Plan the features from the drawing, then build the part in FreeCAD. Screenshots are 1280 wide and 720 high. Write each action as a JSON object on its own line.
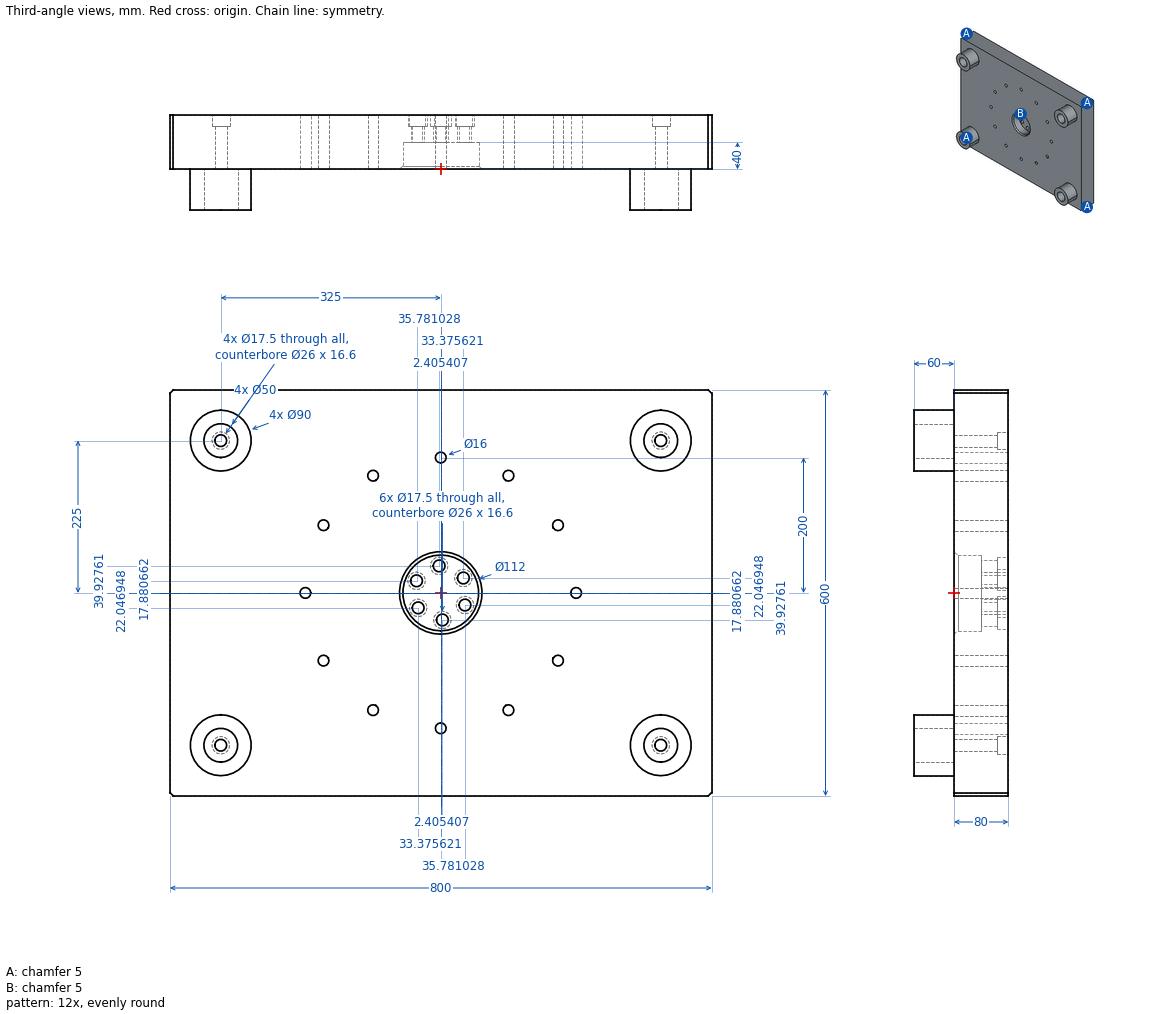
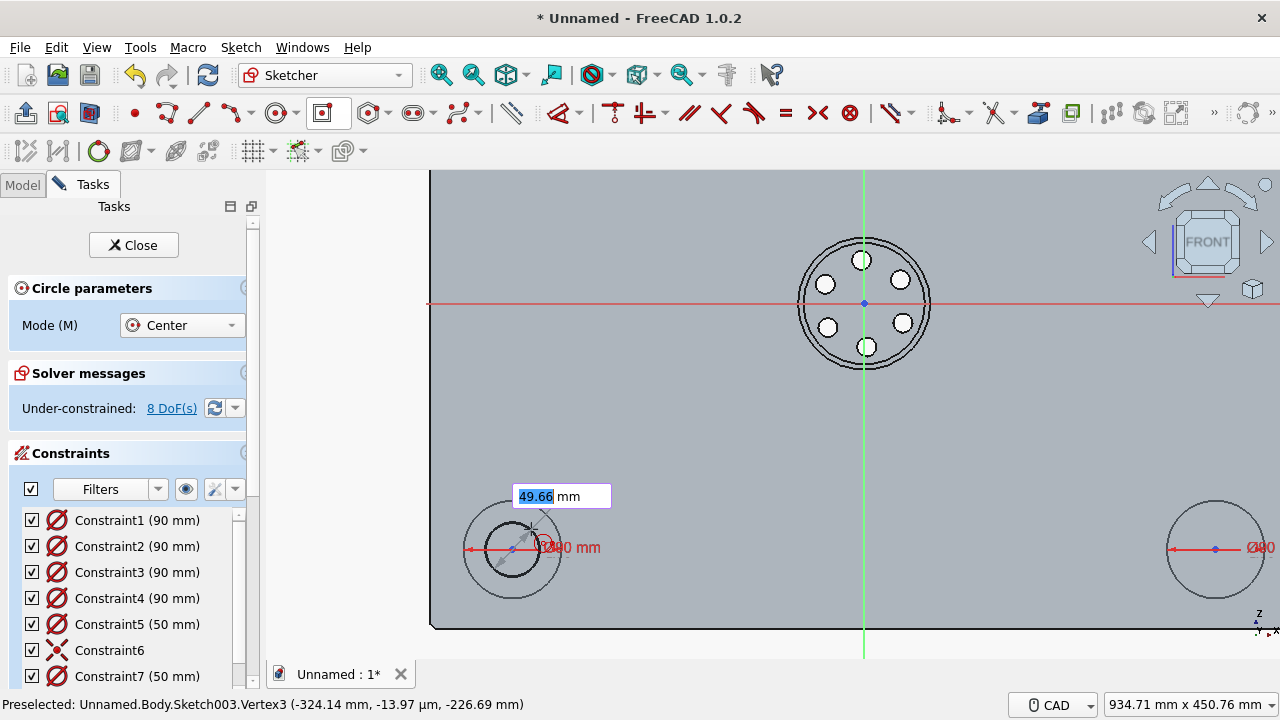
{"action": "type", "text": "50"}
{"action": "key", "text": "Return"}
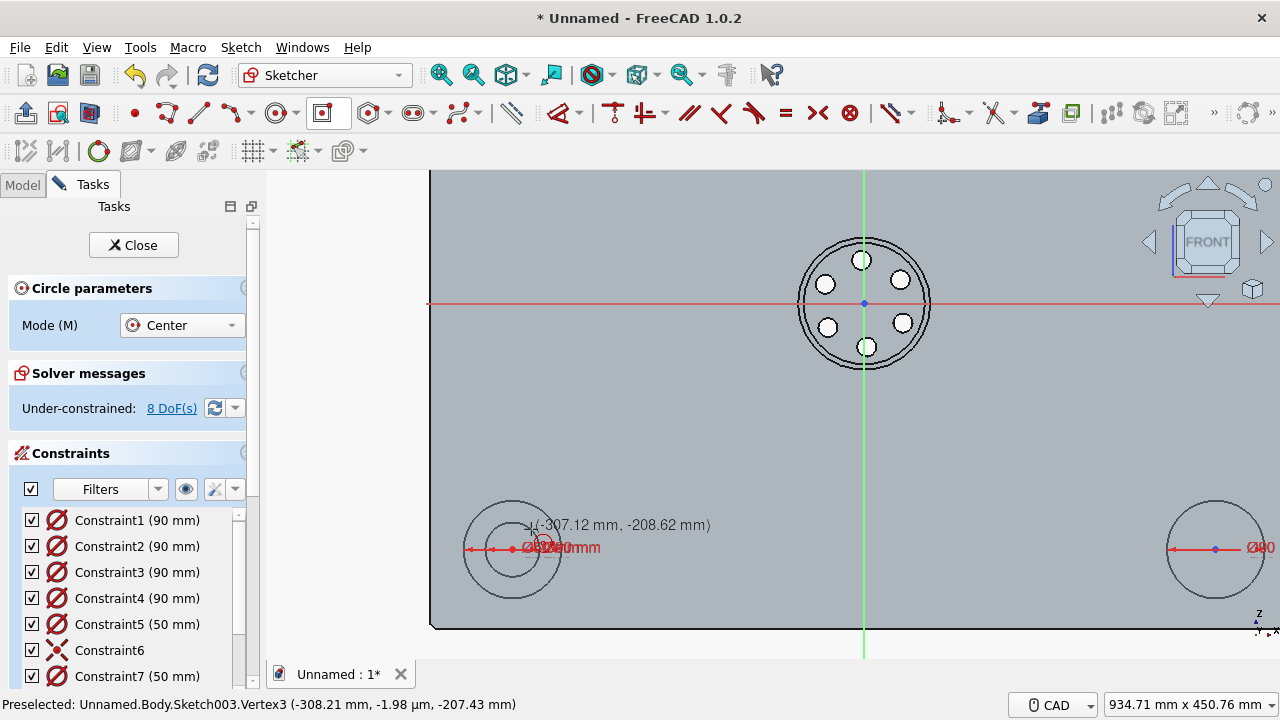
{"action": "scroll", "coordinate": [510, 549], "scroll_direction": "down", "scroll_amount": 3}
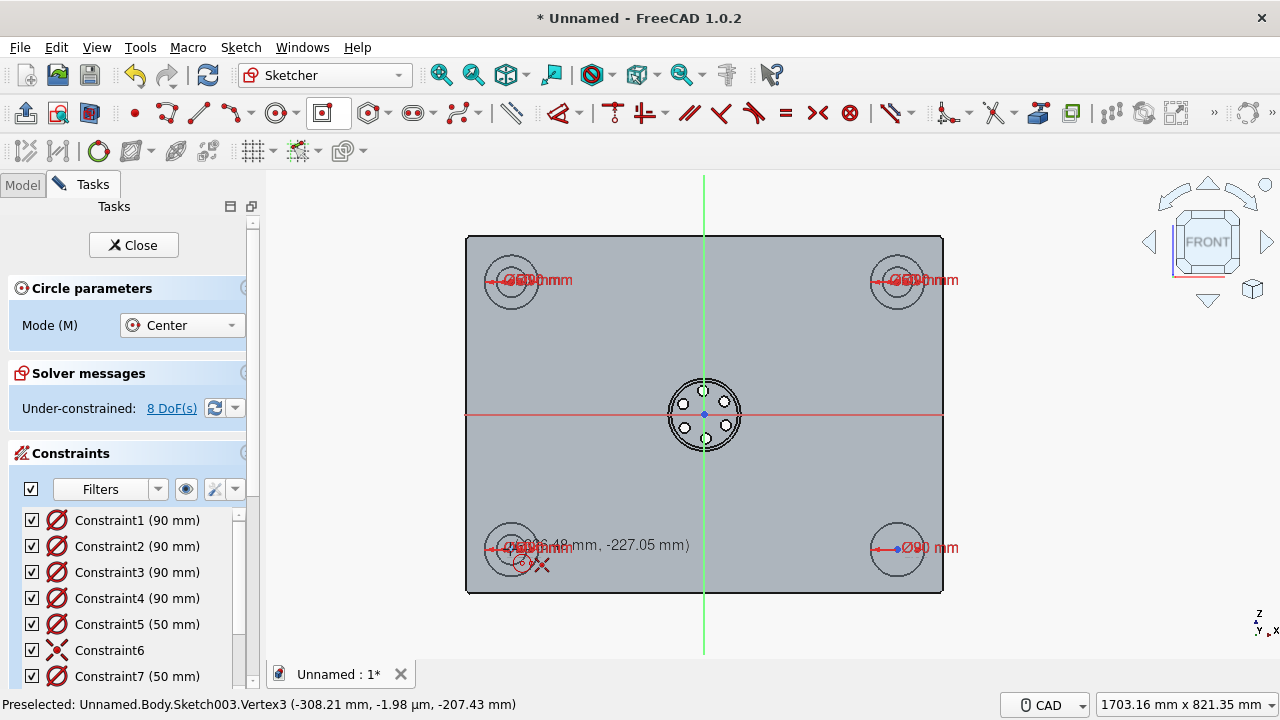
{"action": "scroll", "coordinate": [898, 549], "scroll_direction": "up", "scroll_amount": 3}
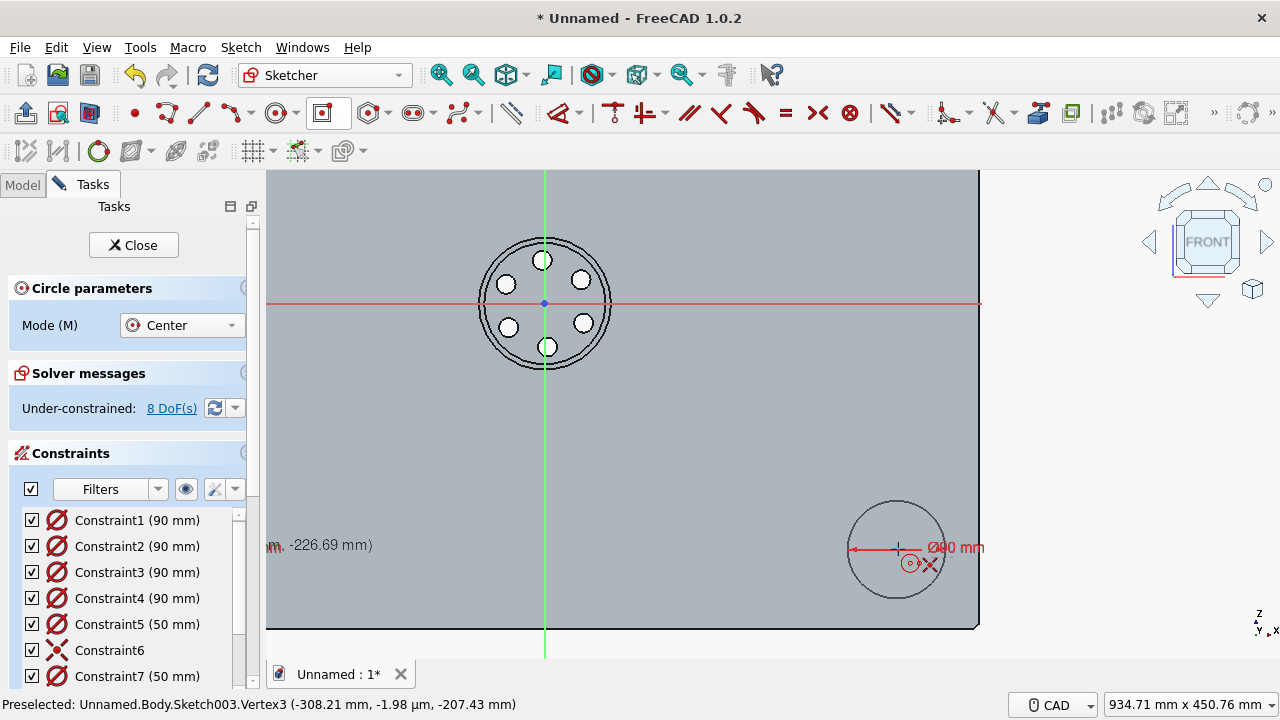
{"action": "left_click", "coordinate": [897, 550]}
{"action": "mouse_move", "coordinate": [917, 529]}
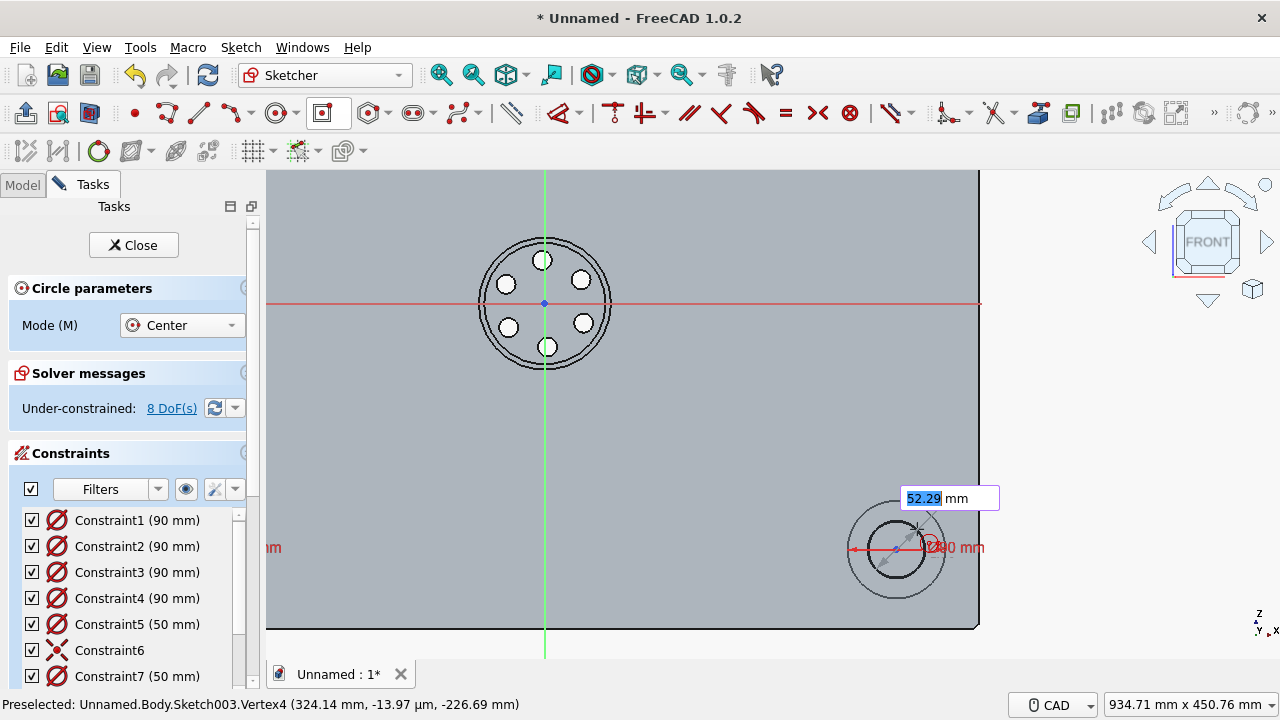
{"action": "type", "text": "50"}
{"action": "key", "text": "Return"}
{"action": "key", "text": "Escape"}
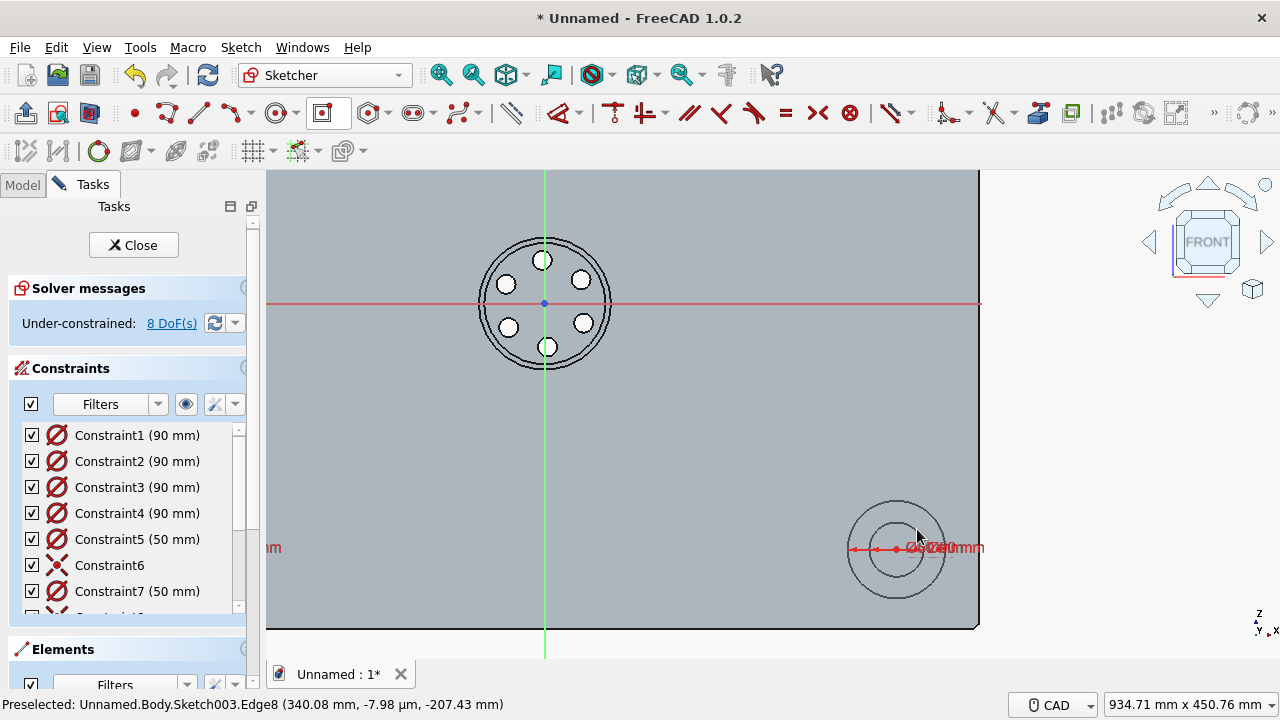
{"action": "scroll", "coordinate": [899, 549], "scroll_direction": "down", "scroll_amount": 3}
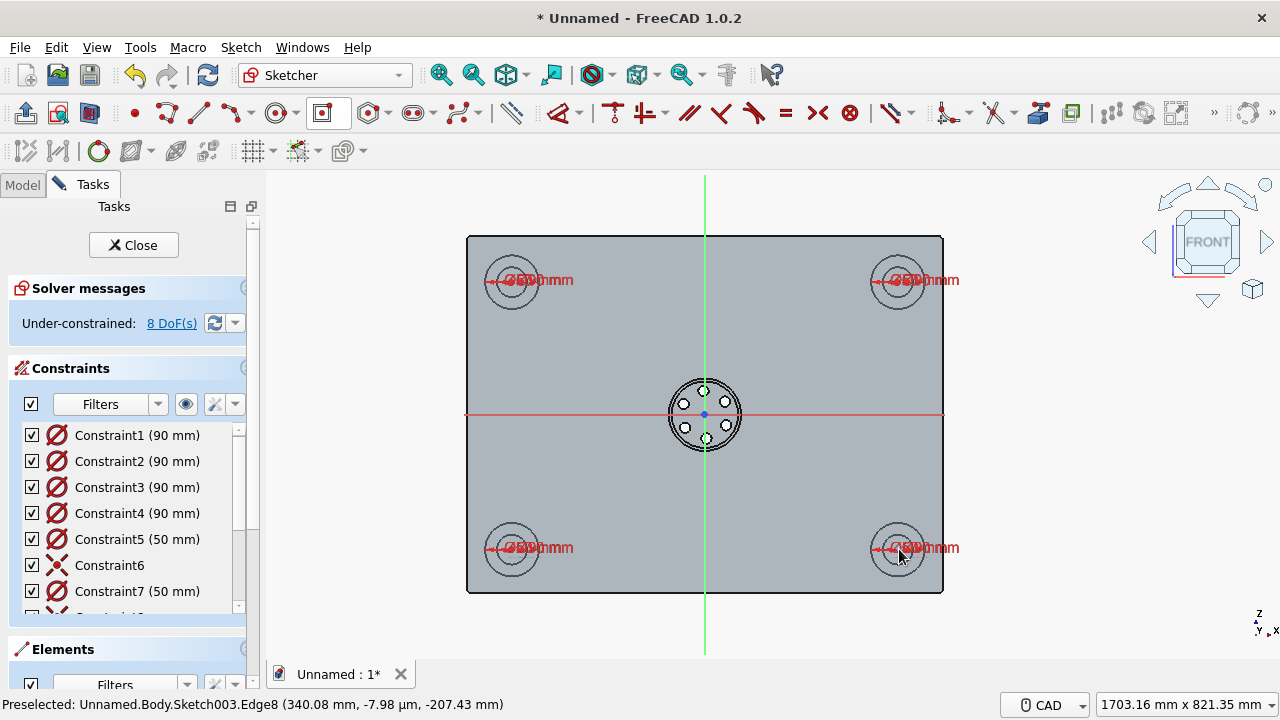
{"action": "left_click", "coordinate": [512, 282]}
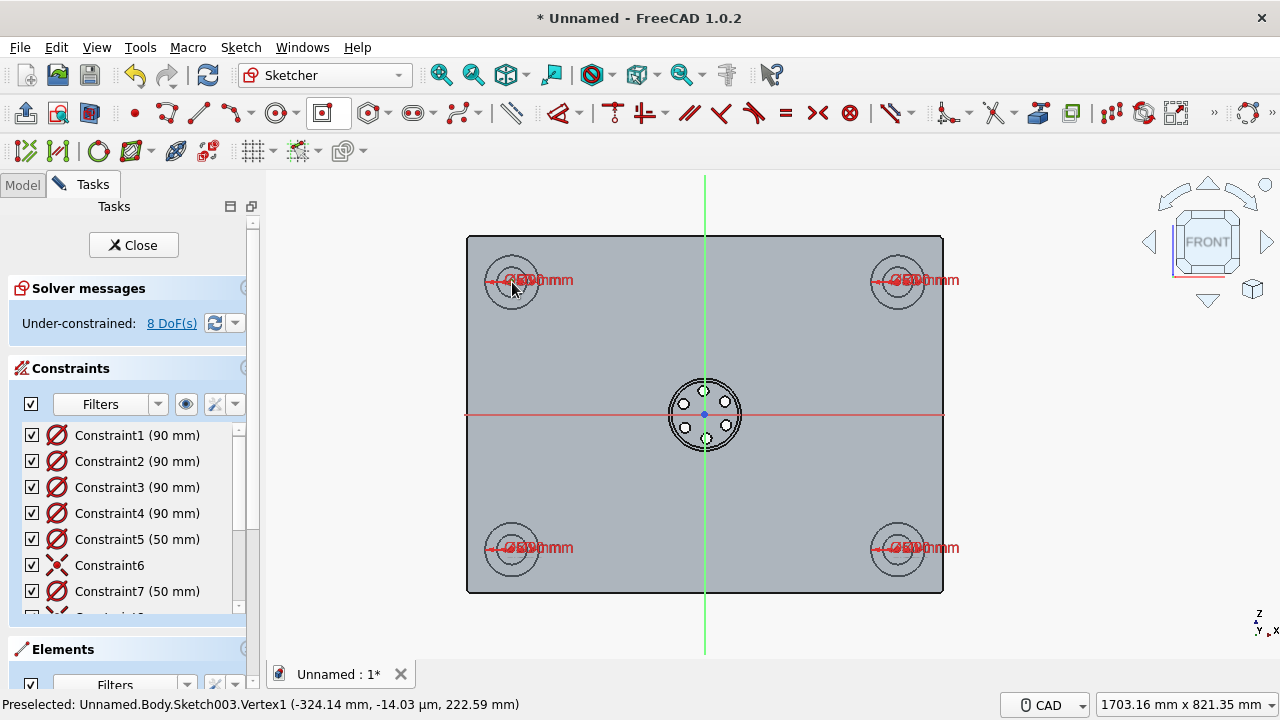
{"action": "left_click", "coordinate": [898, 282]}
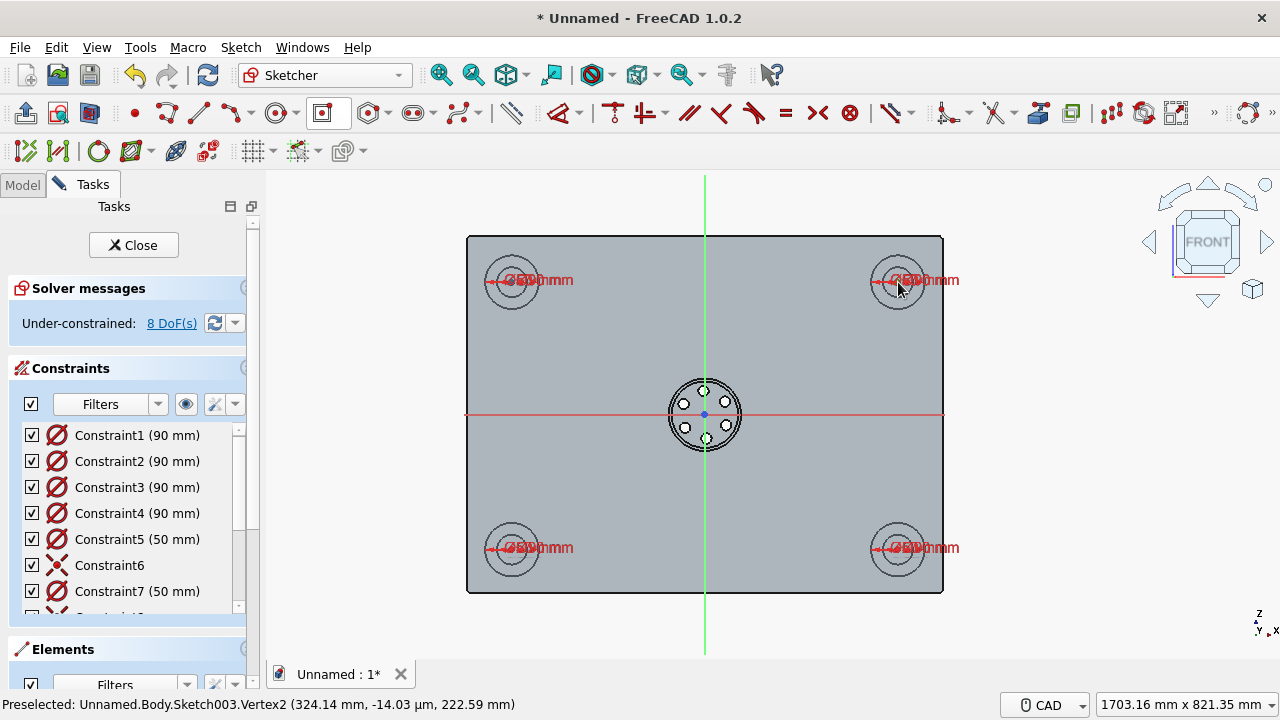
{"action": "left_click", "coordinate": [705, 600]}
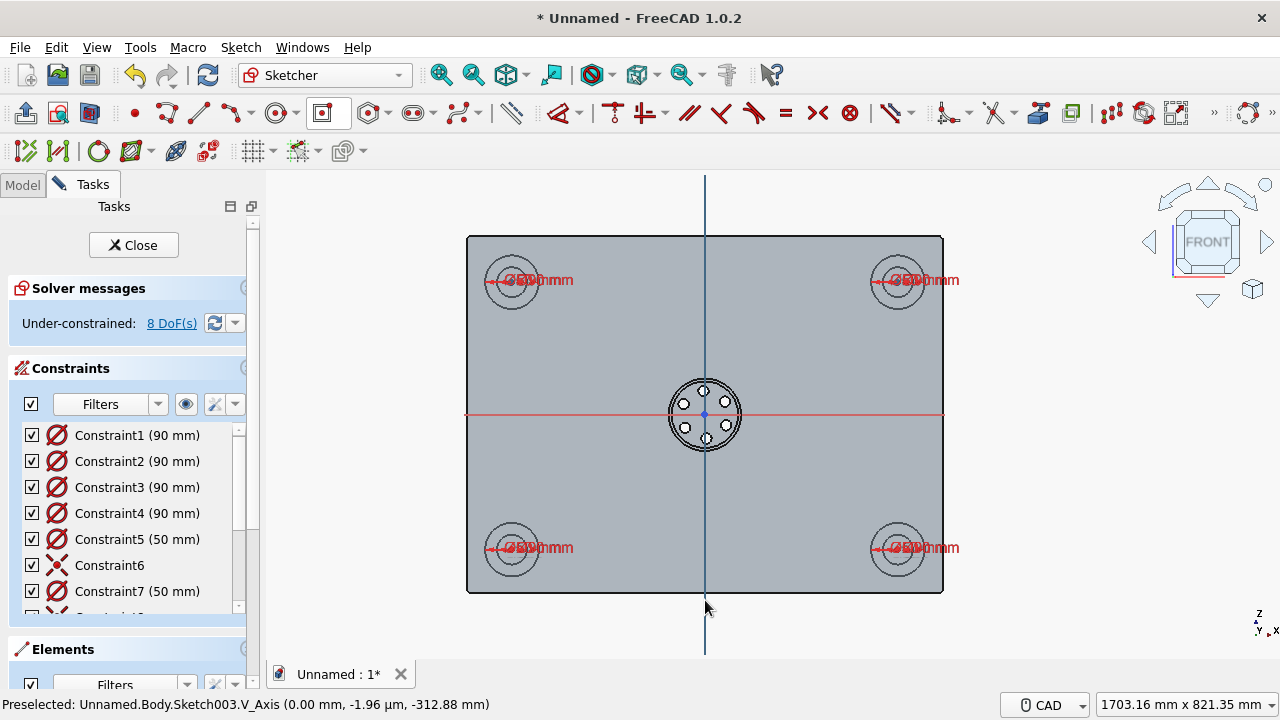
{"action": "key", "text": "s"}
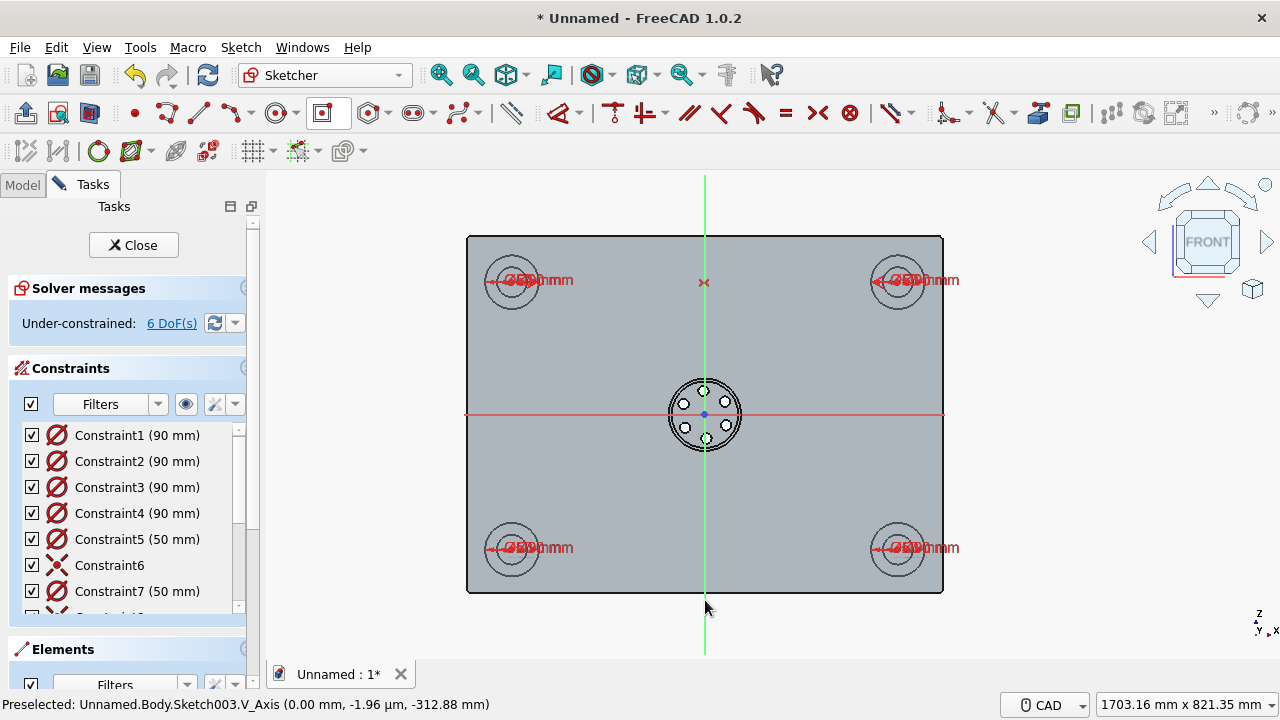
{"action": "left_click", "coordinate": [512, 282]}